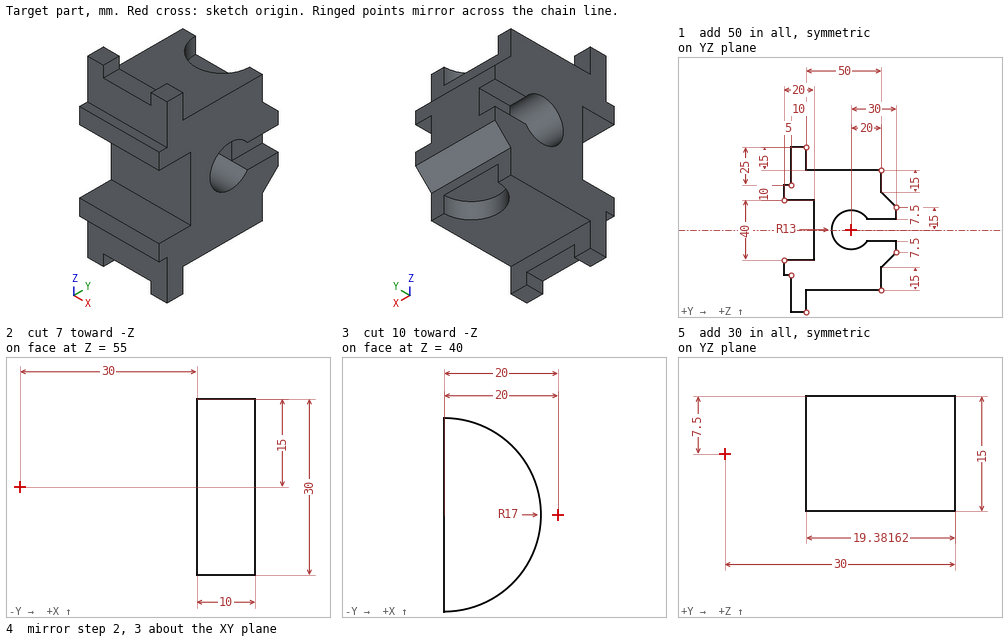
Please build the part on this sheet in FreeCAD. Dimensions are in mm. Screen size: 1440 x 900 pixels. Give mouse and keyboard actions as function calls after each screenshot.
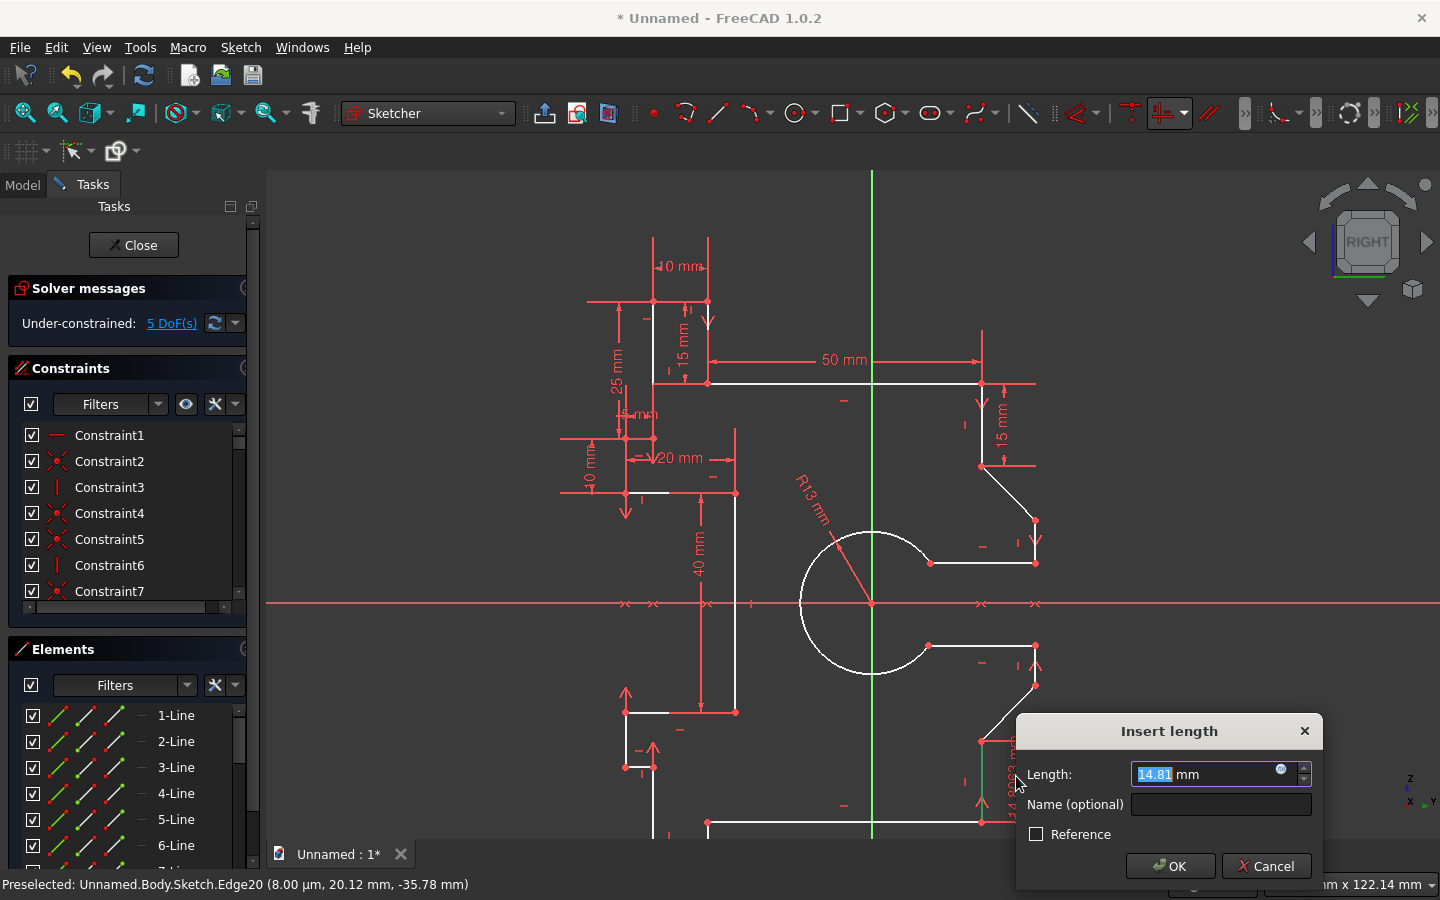
text(15)
key(Return)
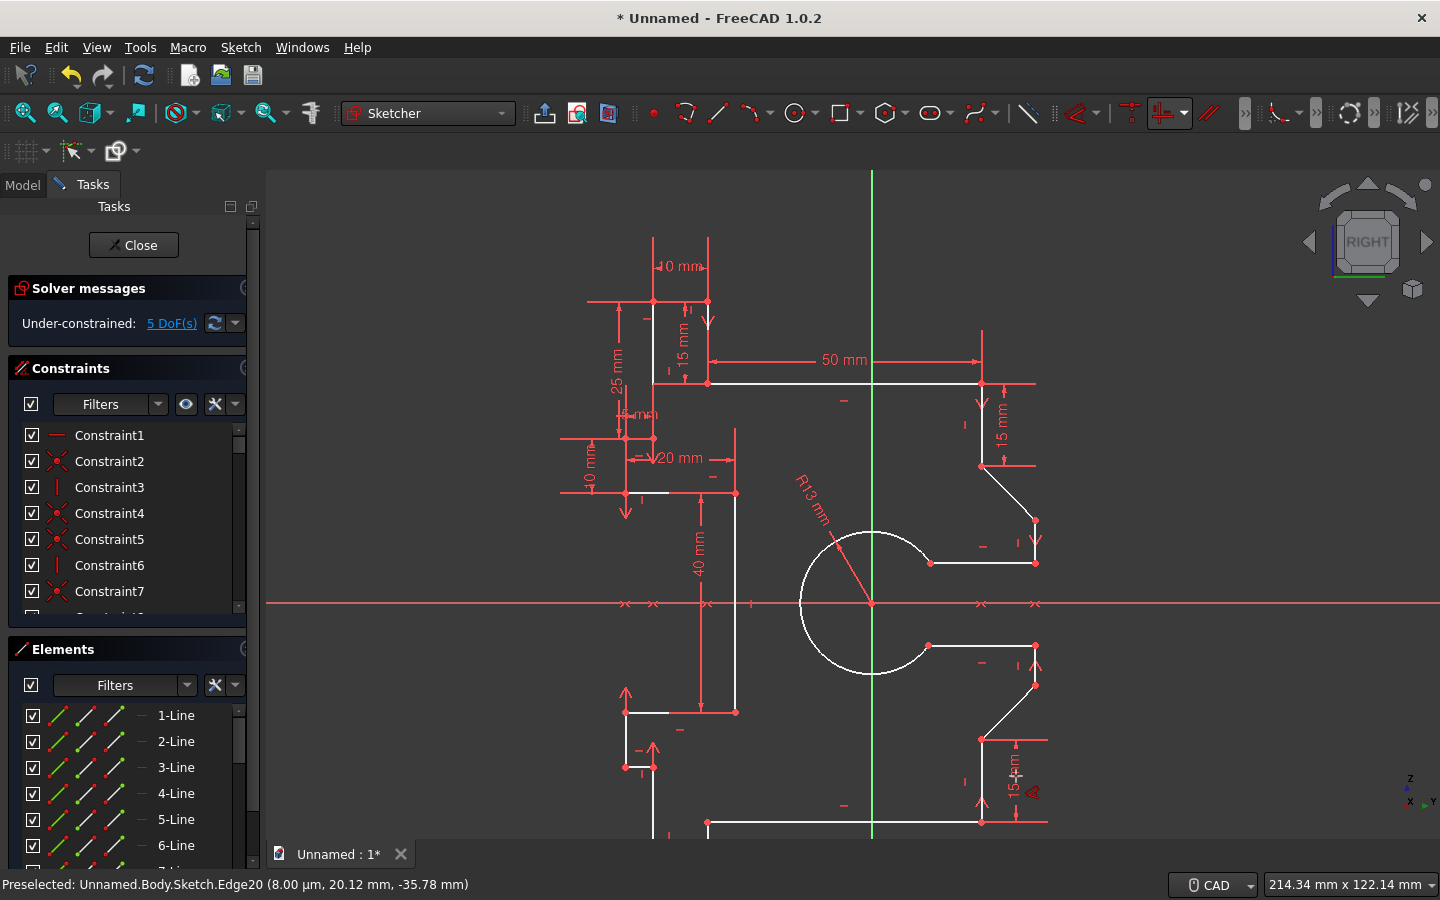
click(1035, 551)
click(1069, 542)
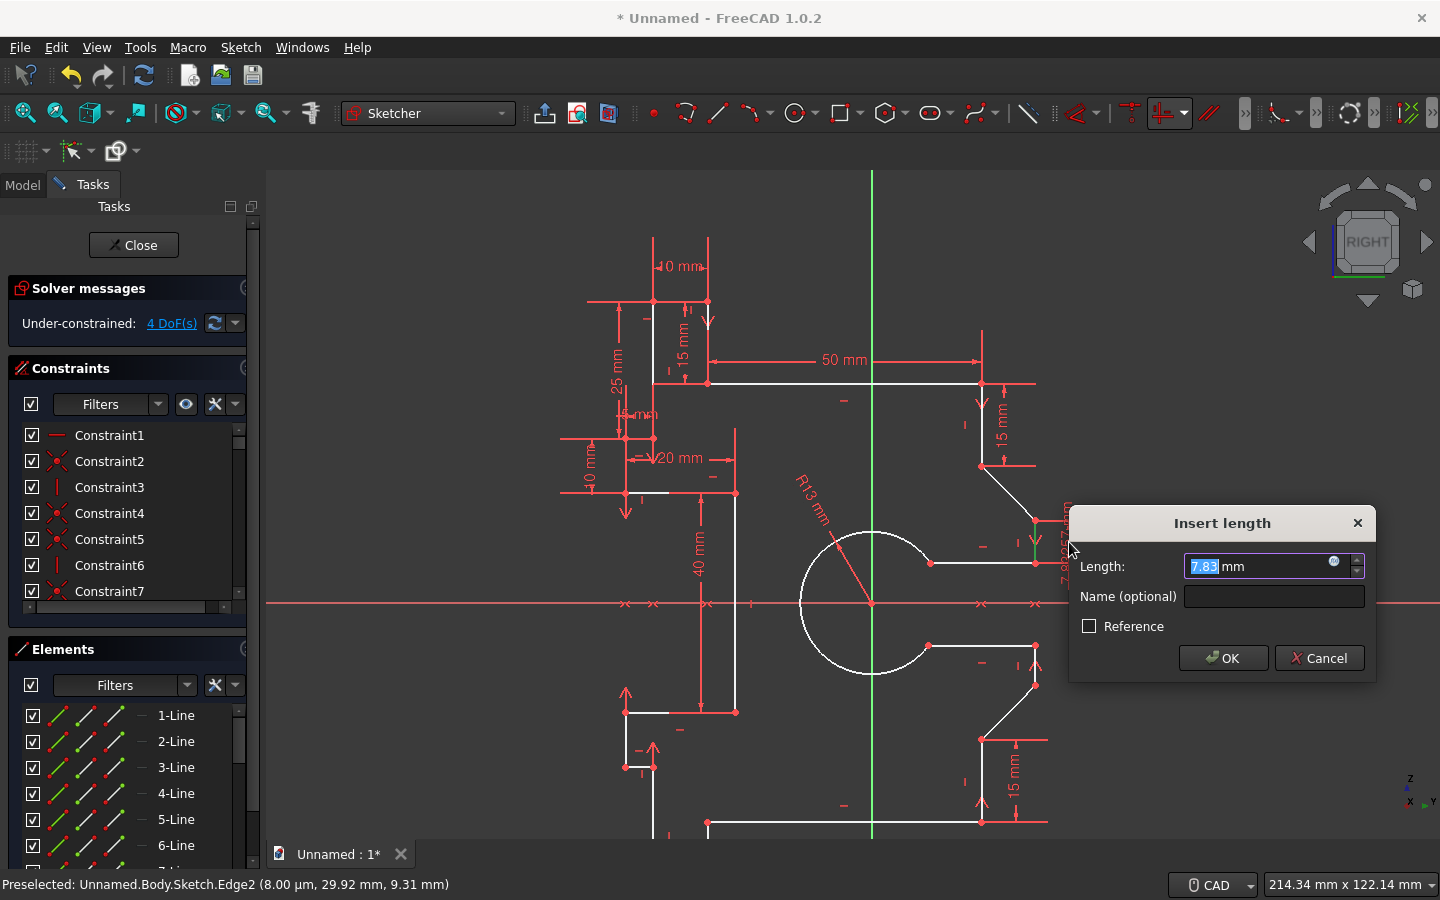
text(7.5)
key(Return)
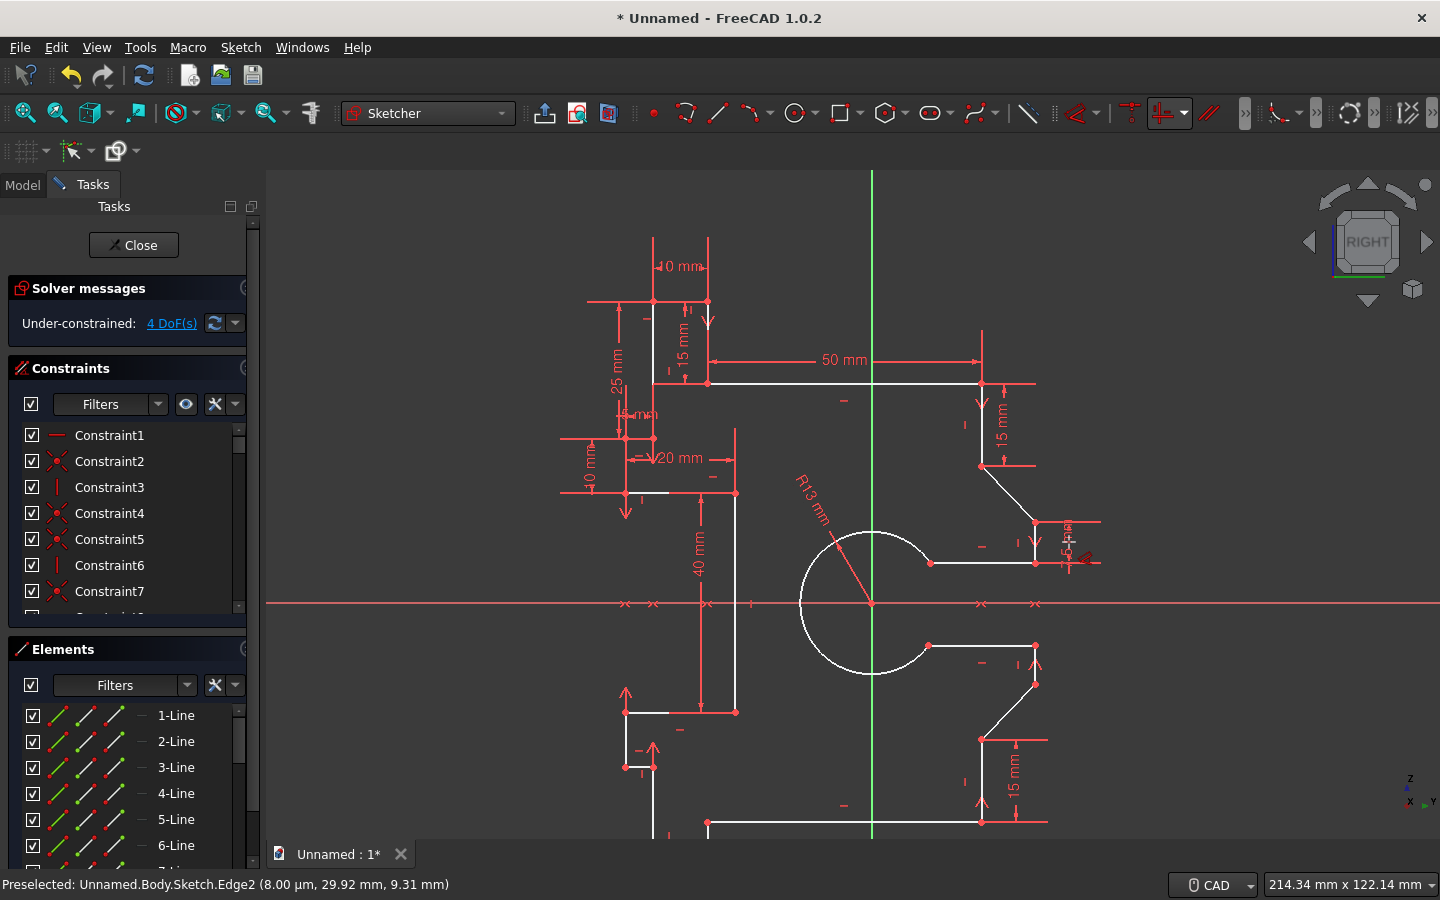
click(1035, 672)
click(1069, 665)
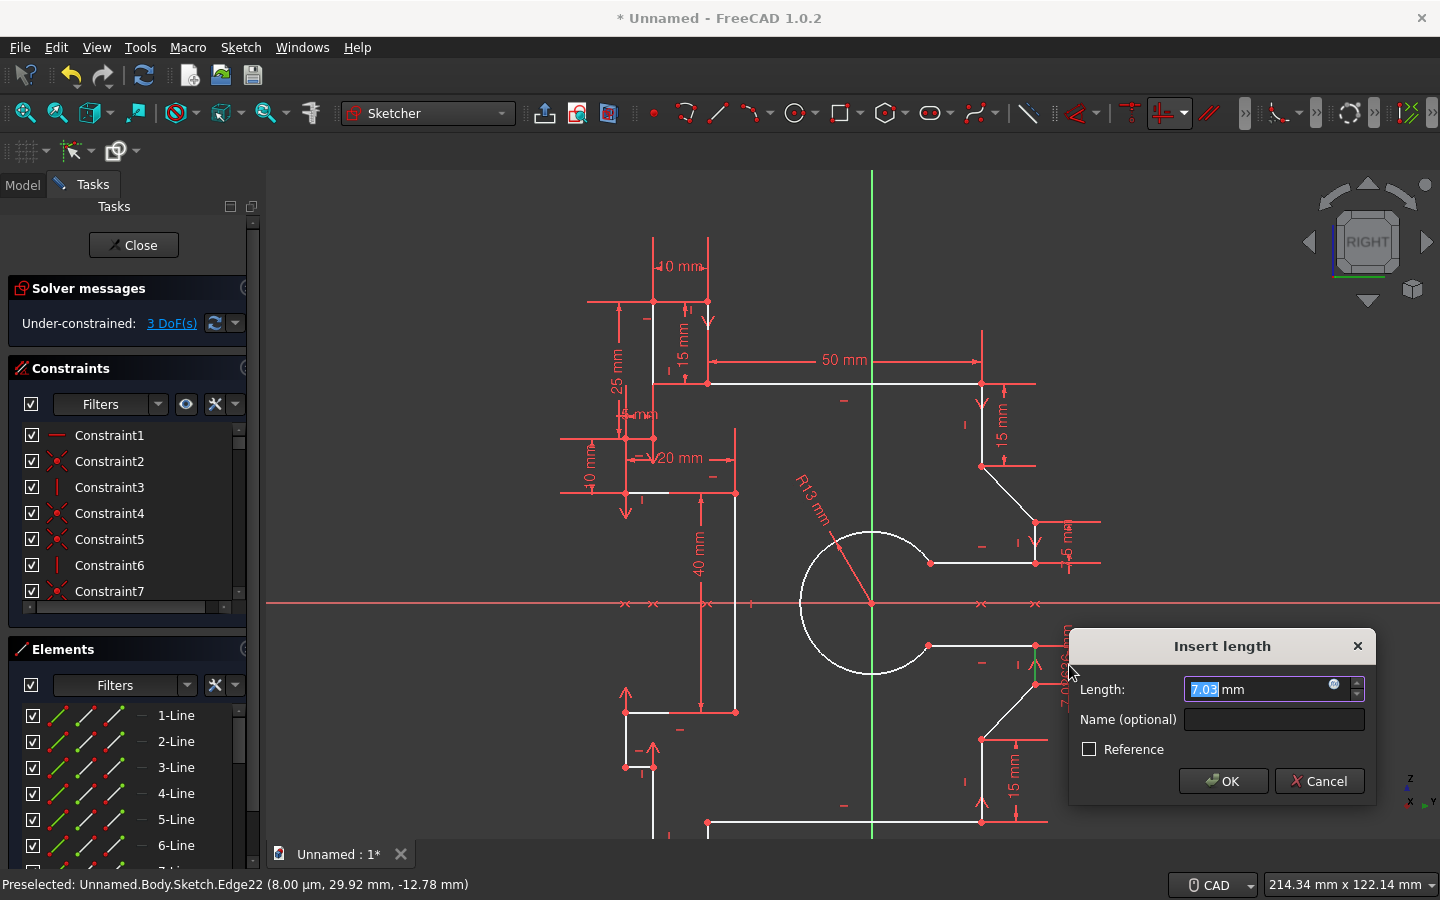
text(7.5)
key(Return)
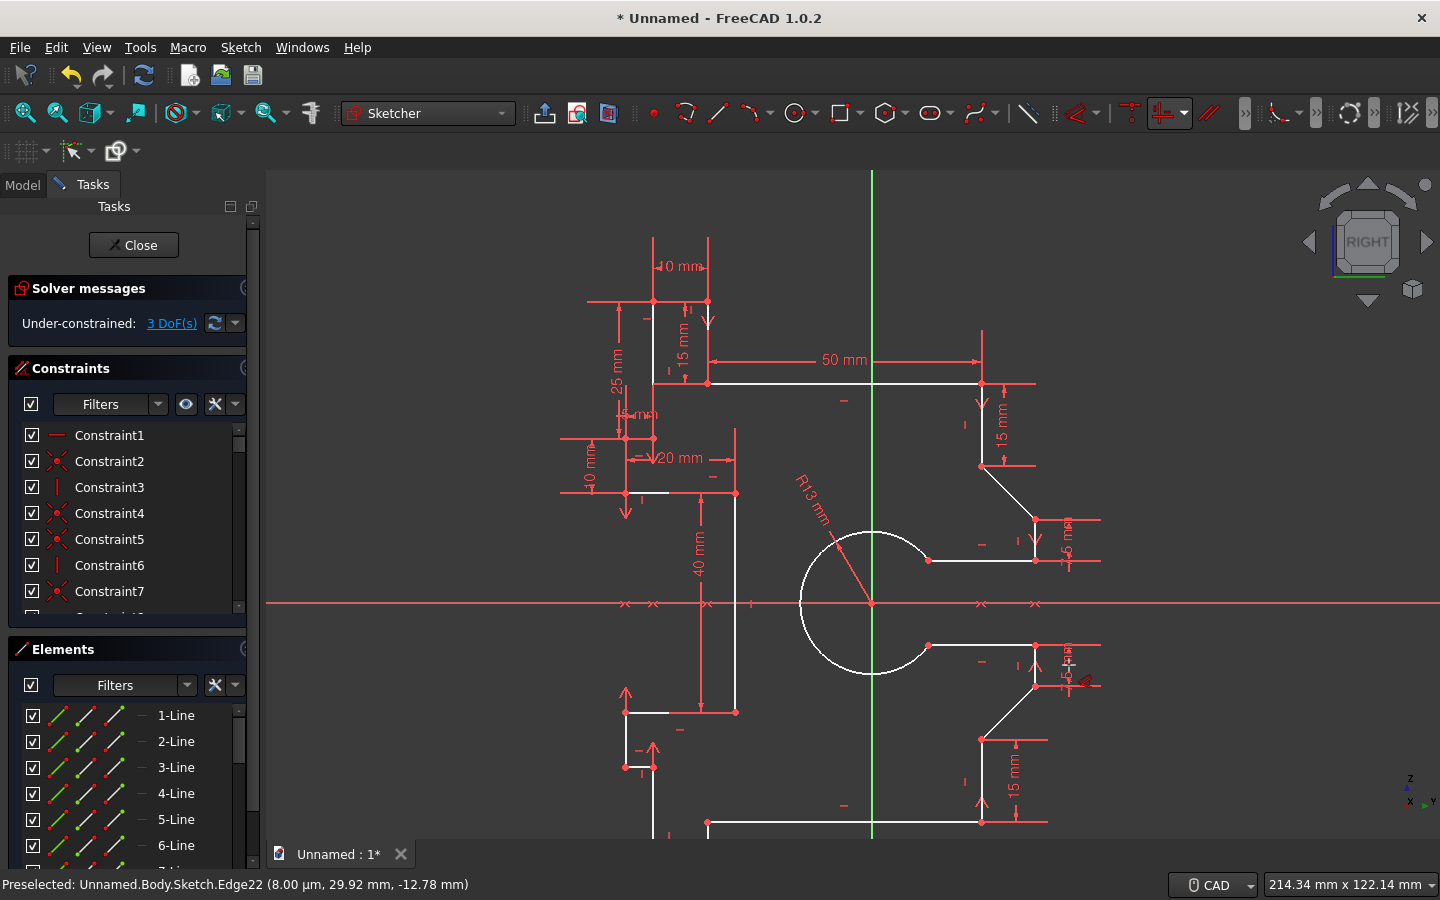
click(1035, 561)
click(953, 527)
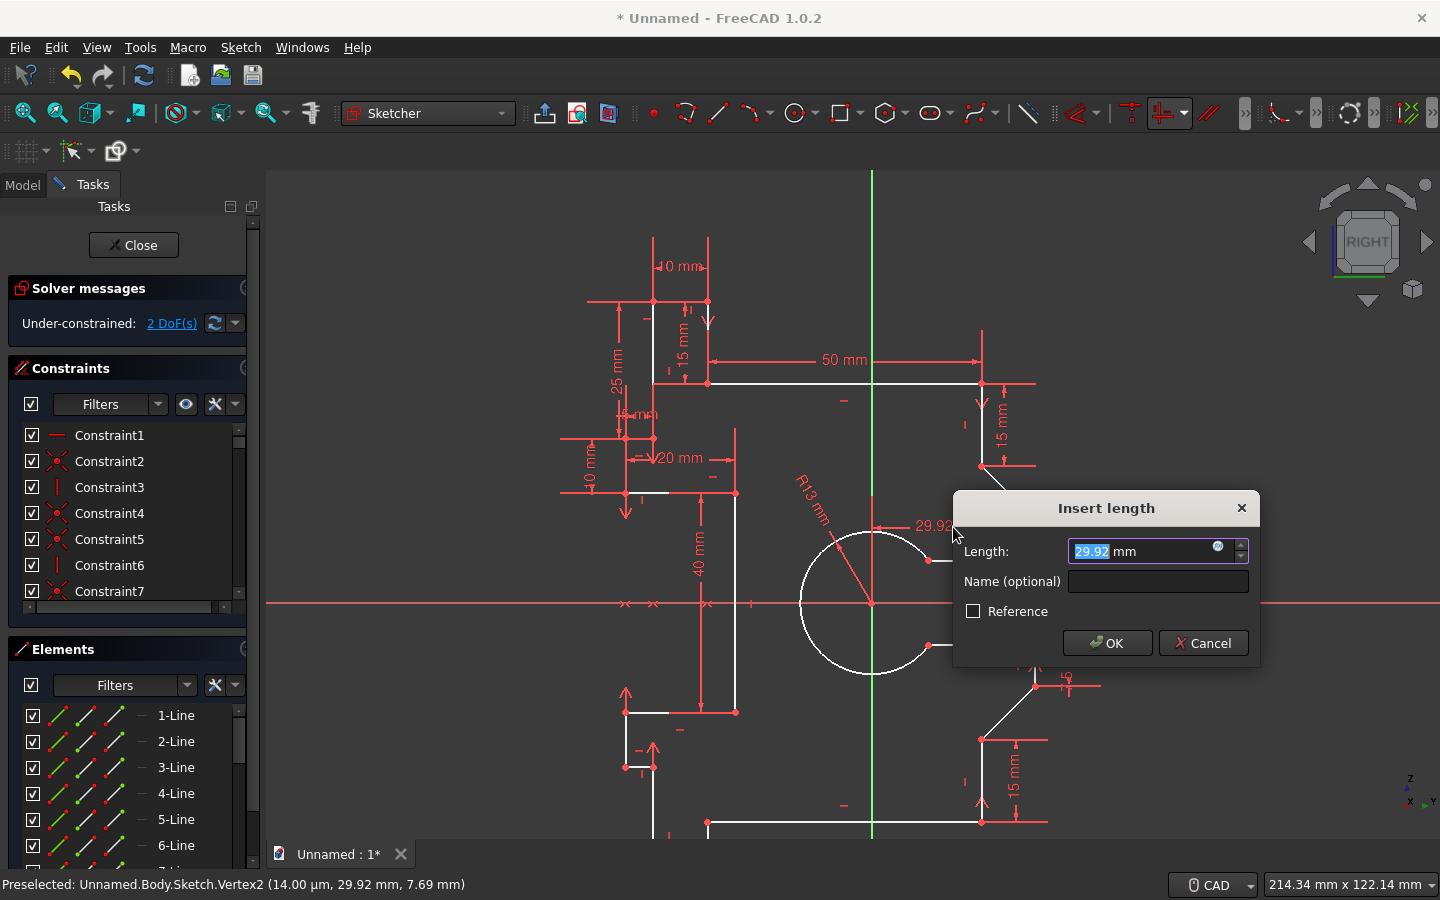
text(30)
key(Return)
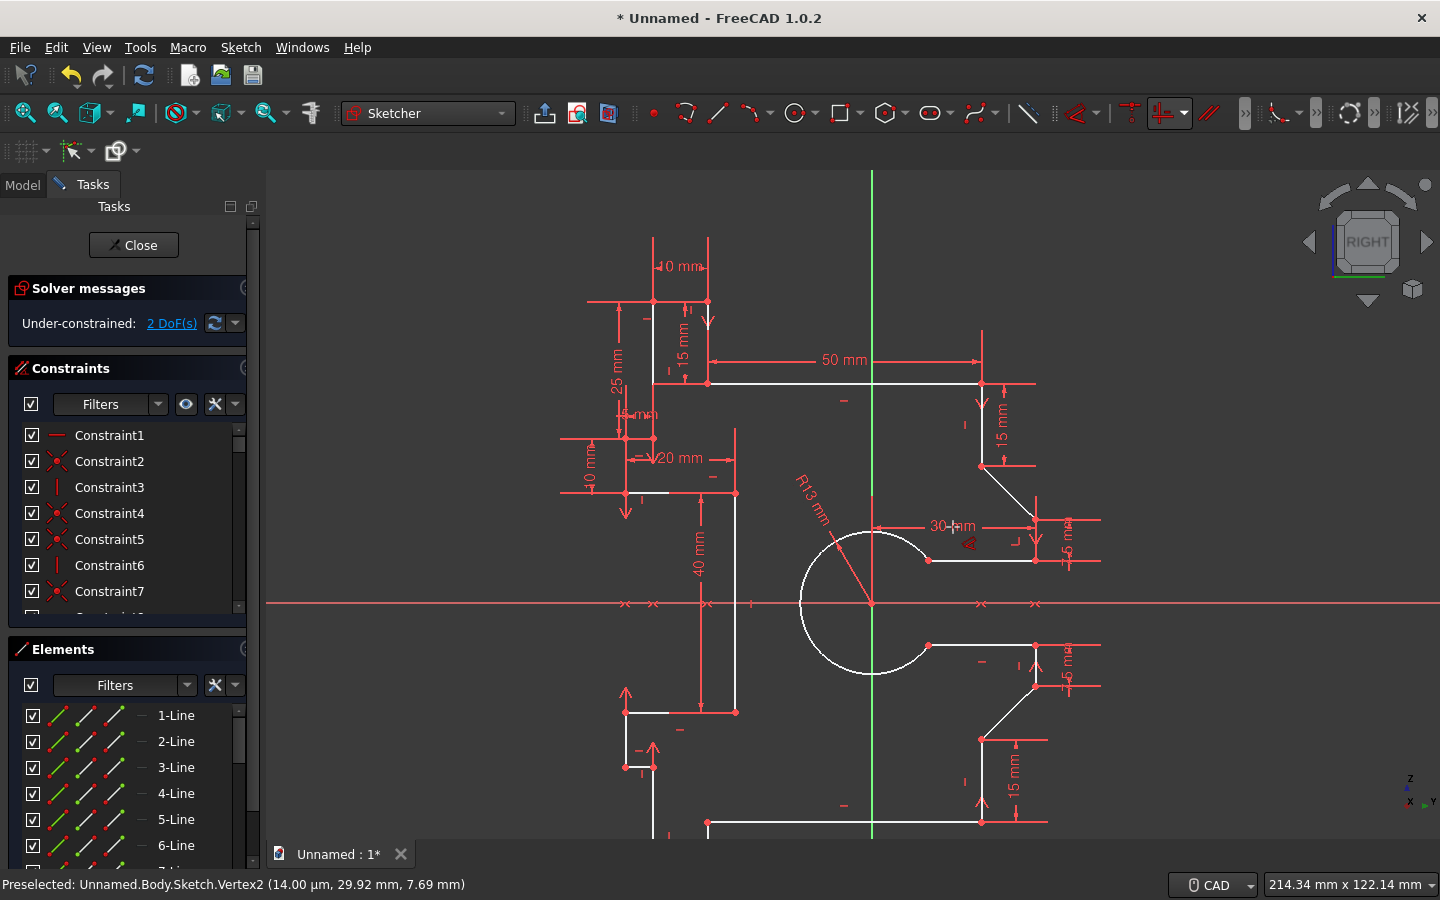
click(1036, 520)
click(1070, 581)